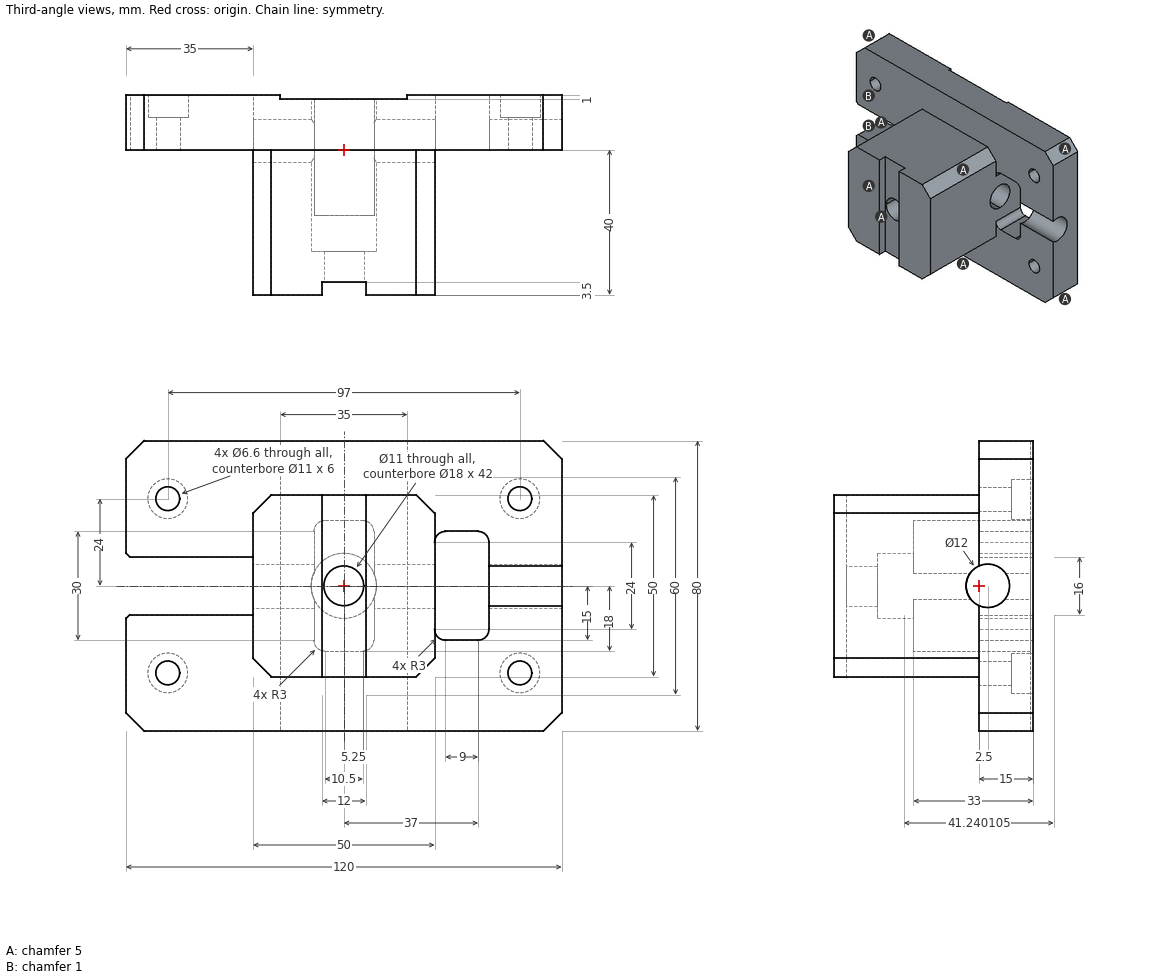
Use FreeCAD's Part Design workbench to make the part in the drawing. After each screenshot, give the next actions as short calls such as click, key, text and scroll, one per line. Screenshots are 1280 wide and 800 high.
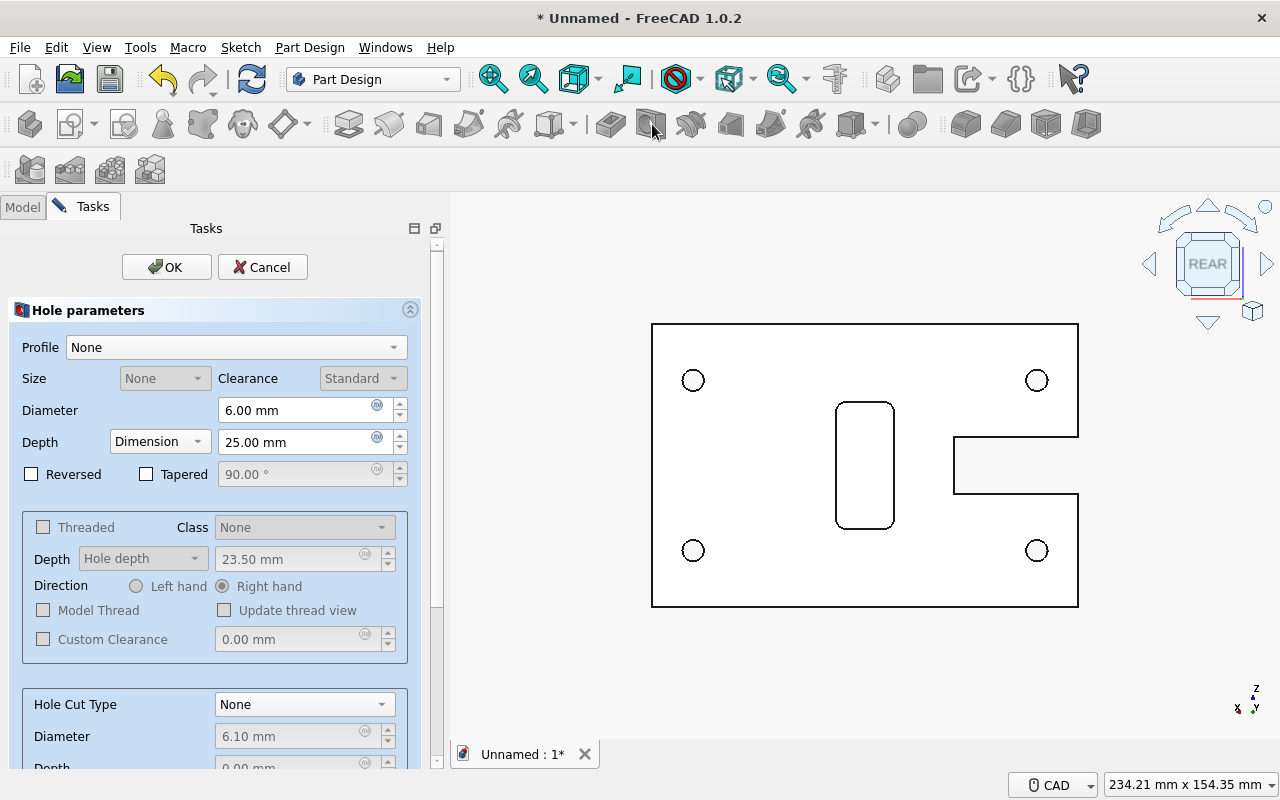
triple_click(305, 410)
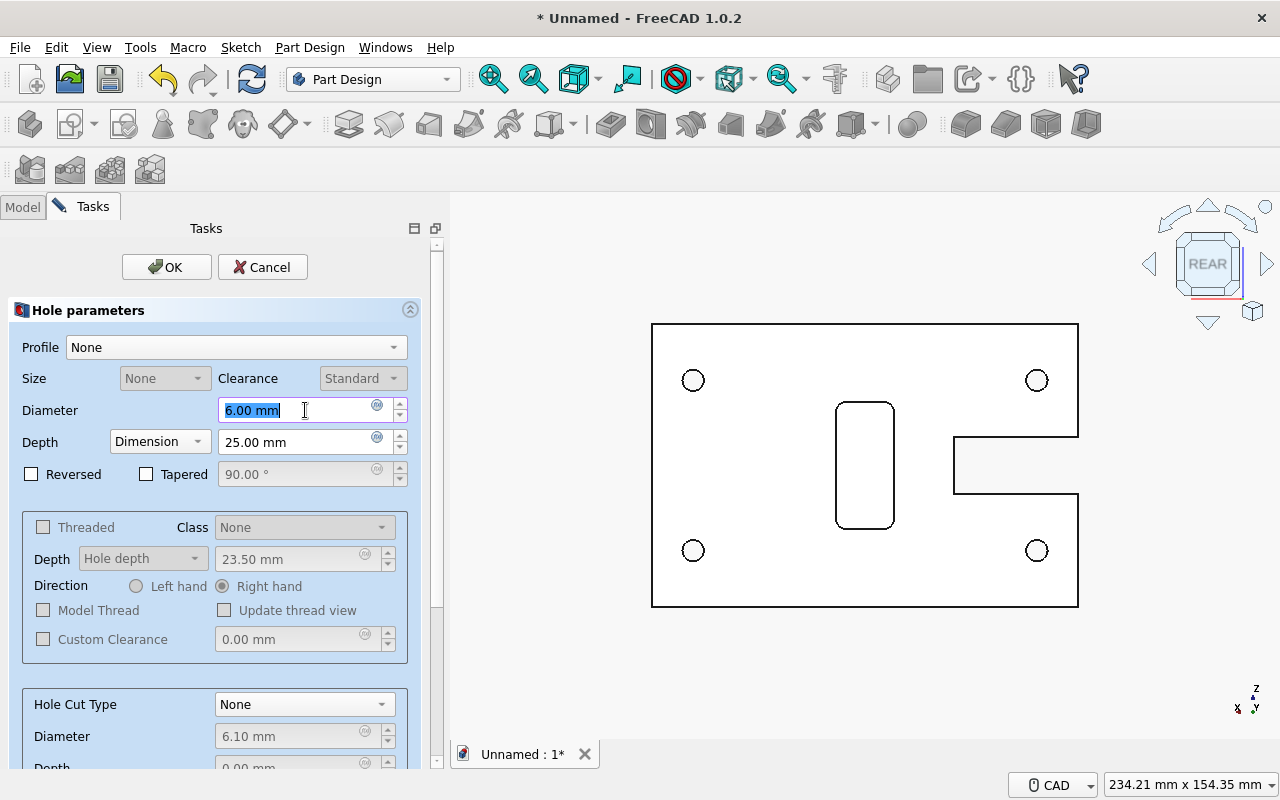
text(6.6)
key(Tab)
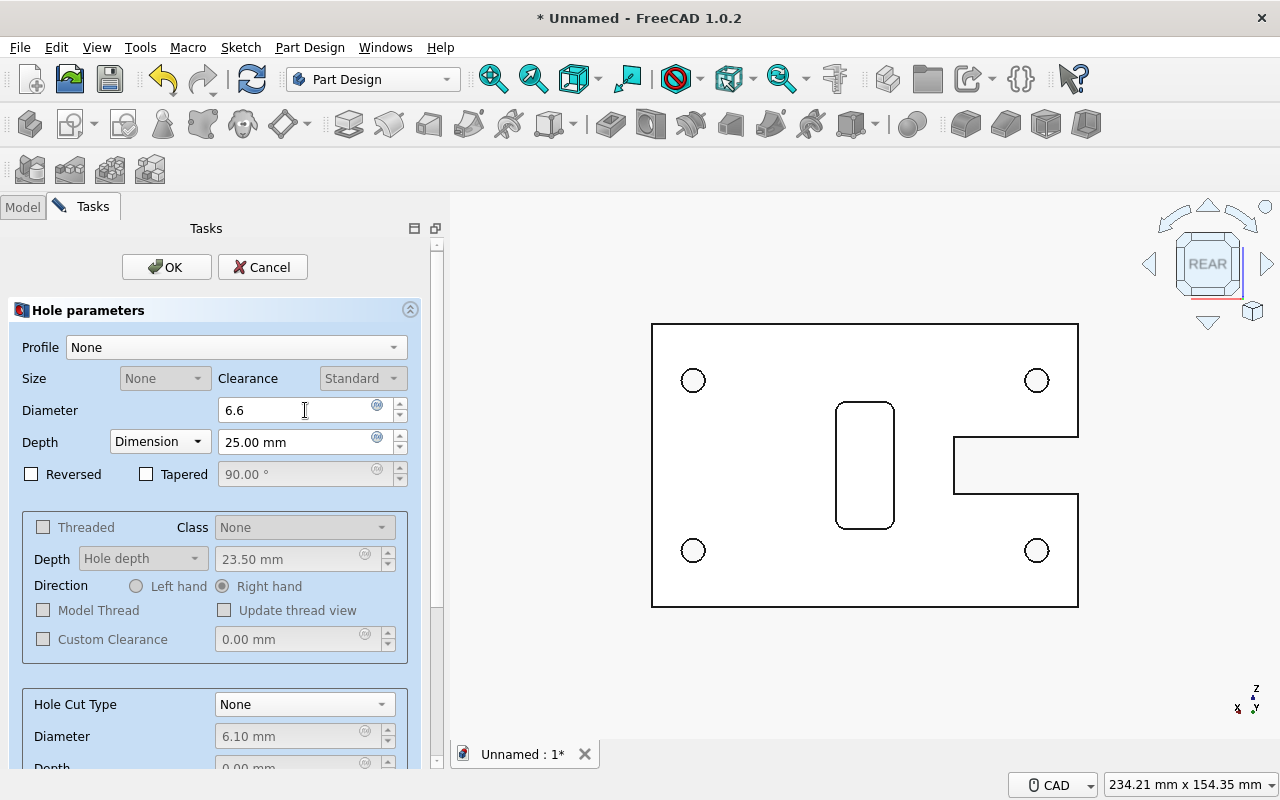
click(161, 442)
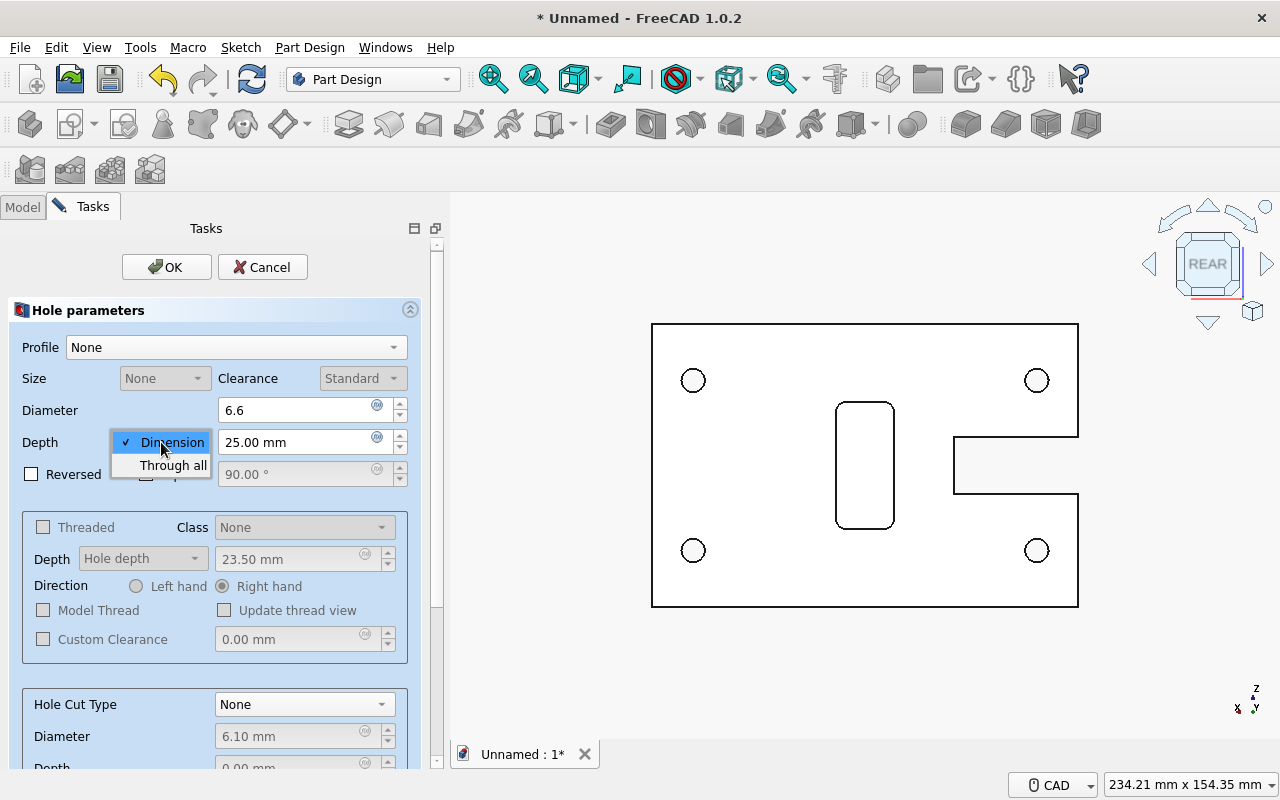
click(160, 466)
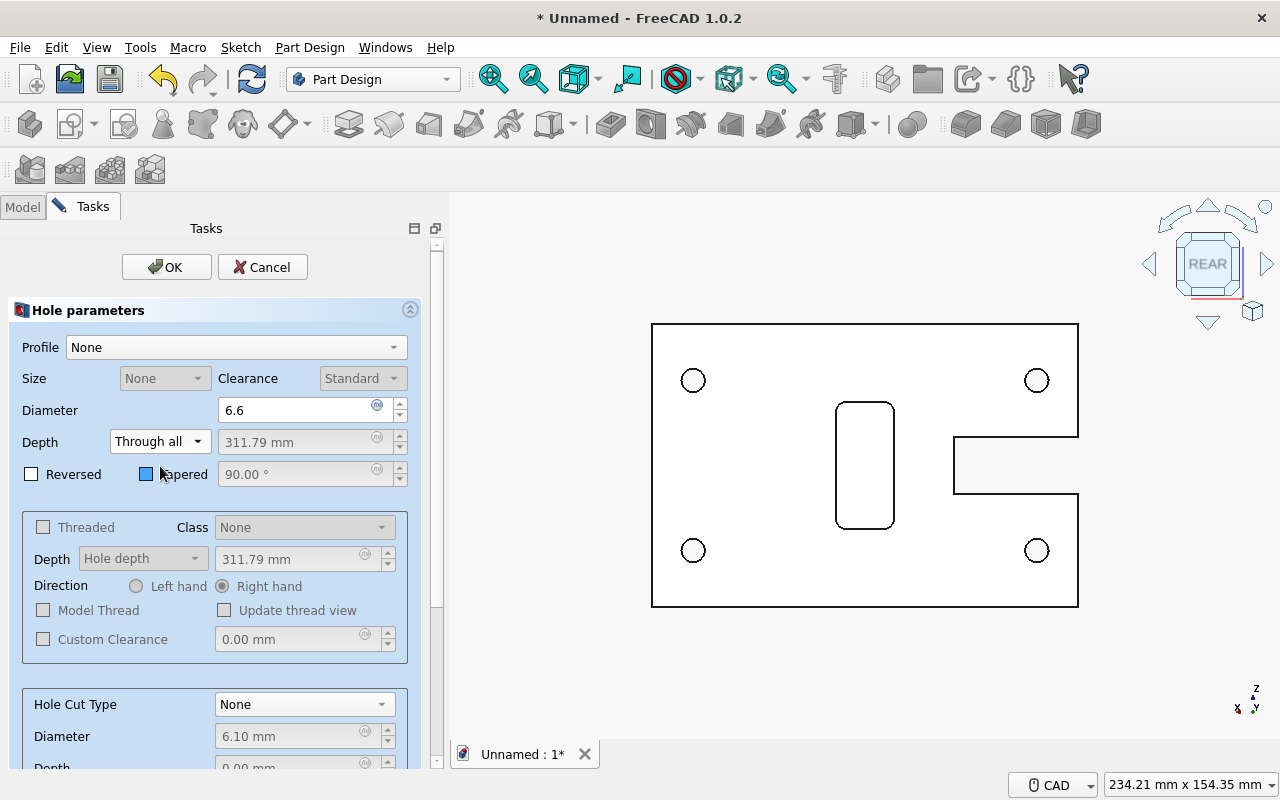
click(306, 704)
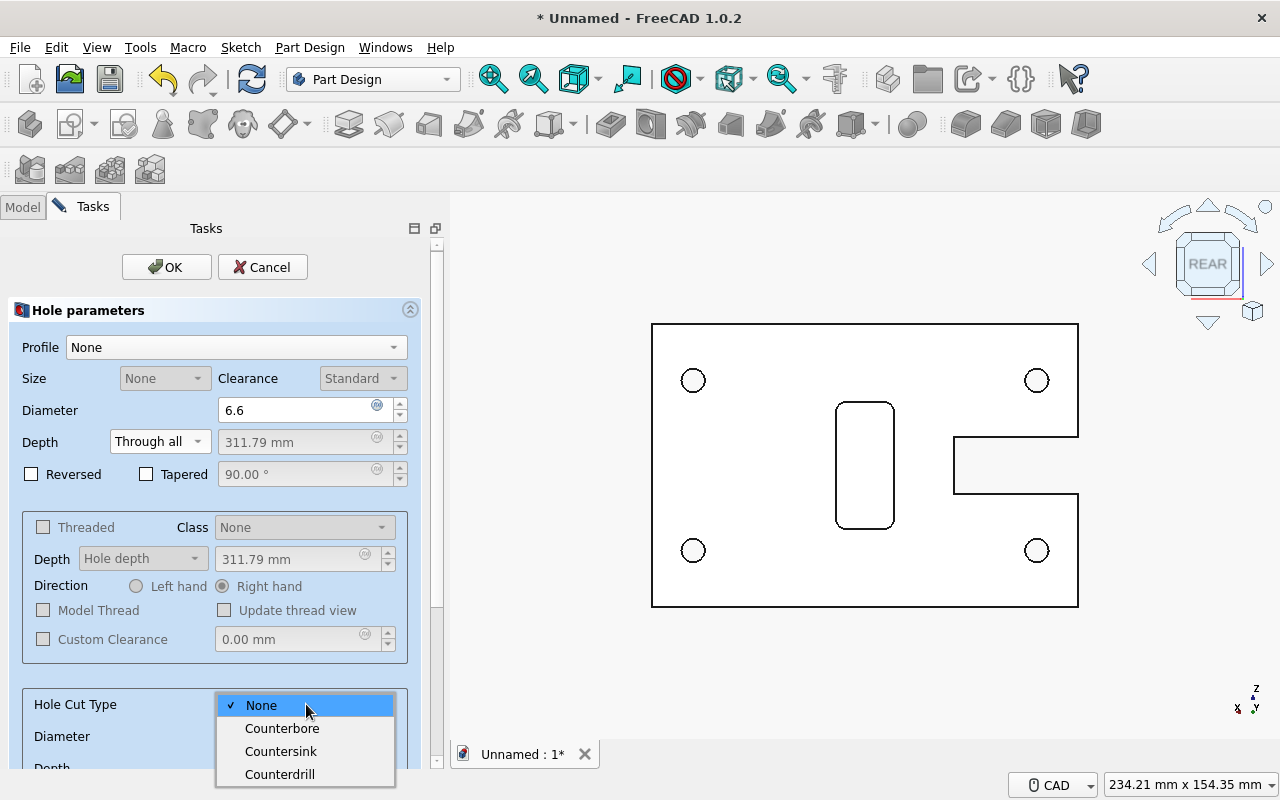
click(304, 728)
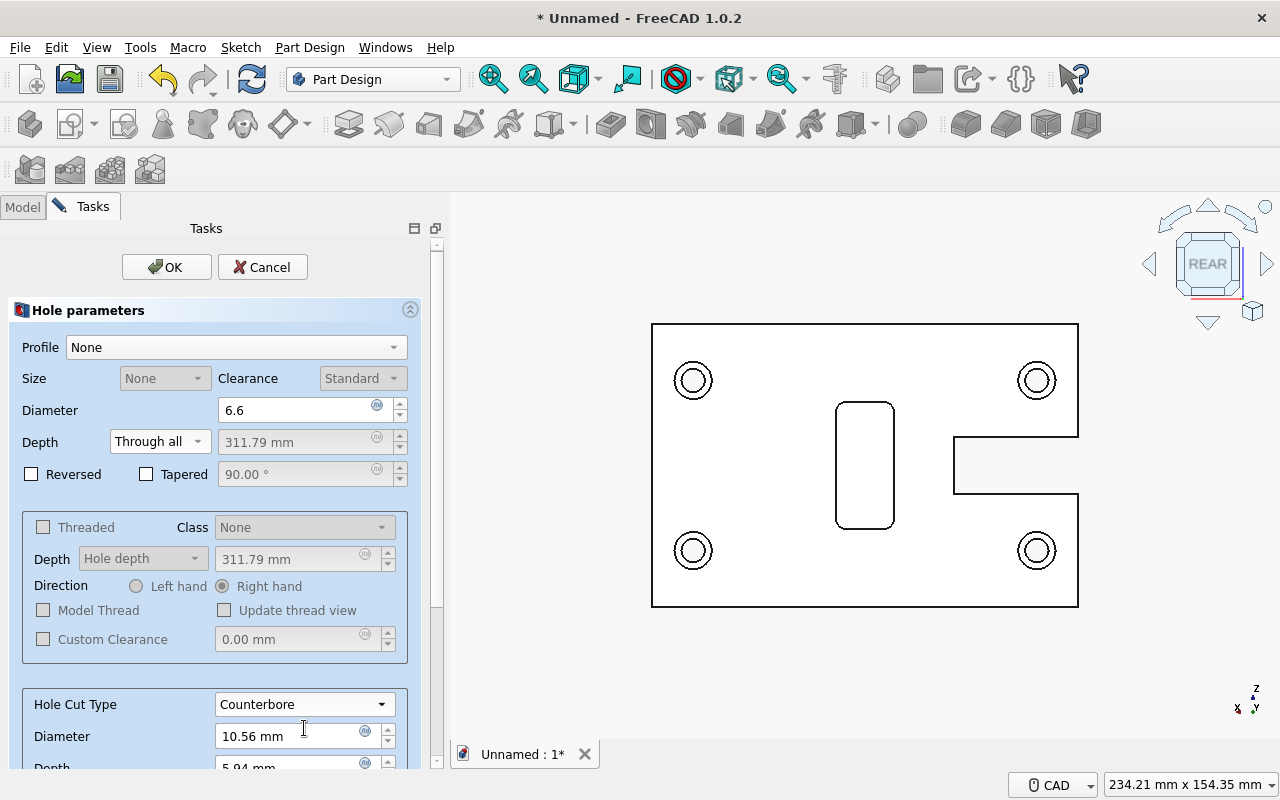
triple_click(298, 736)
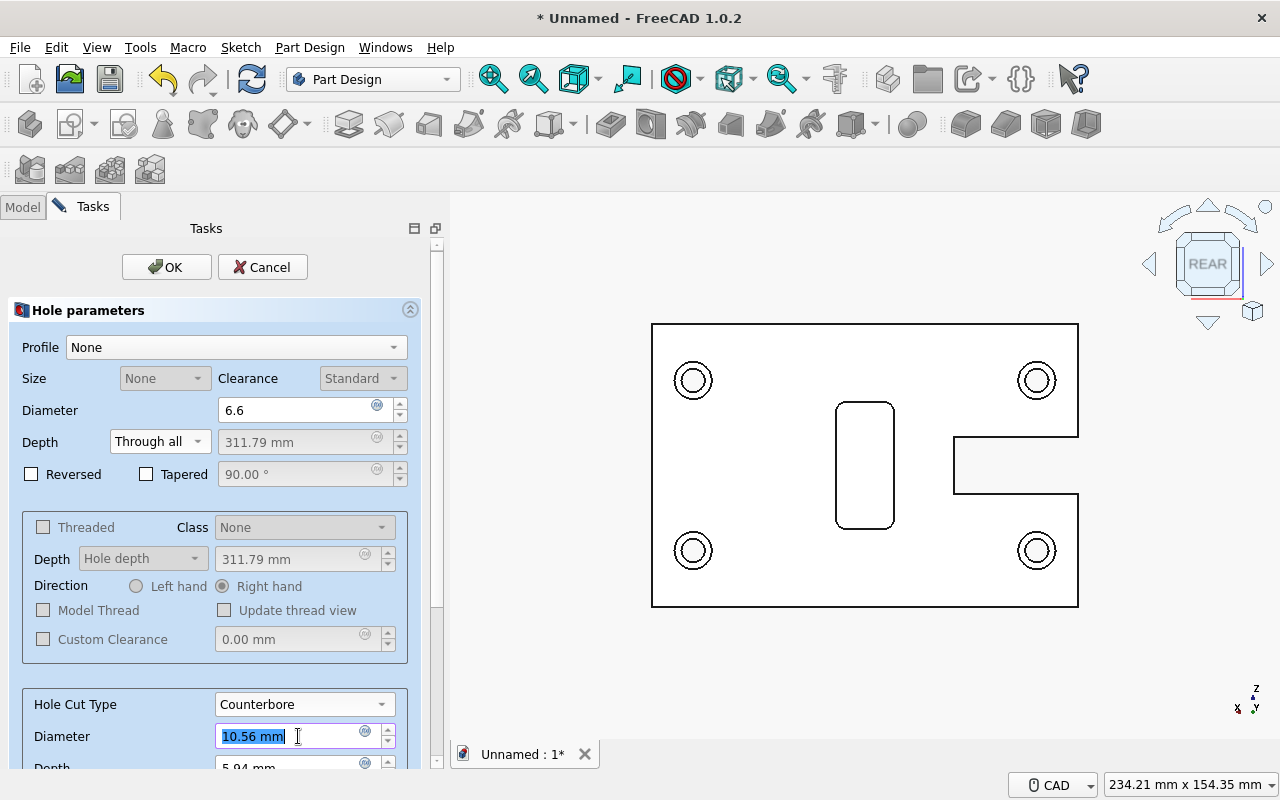
text(11)
key(Tab)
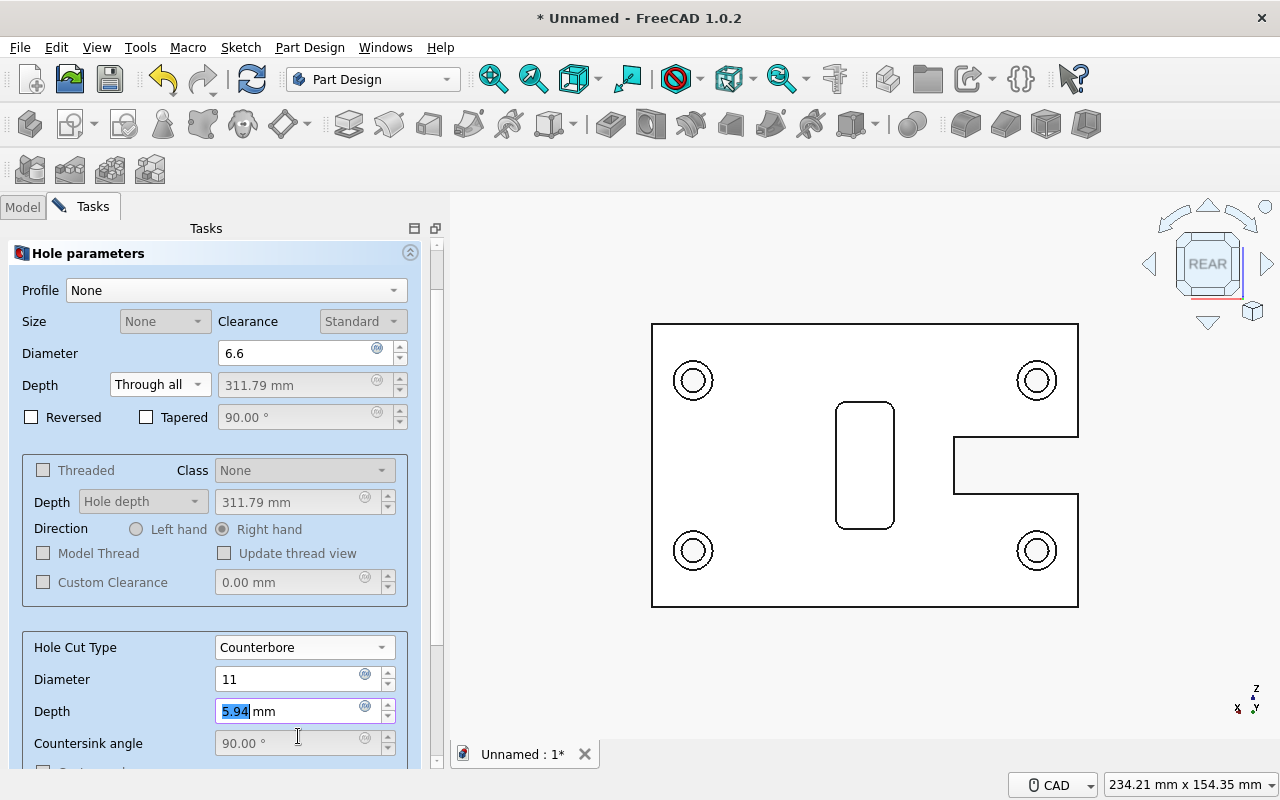
text(6)
key(Tab)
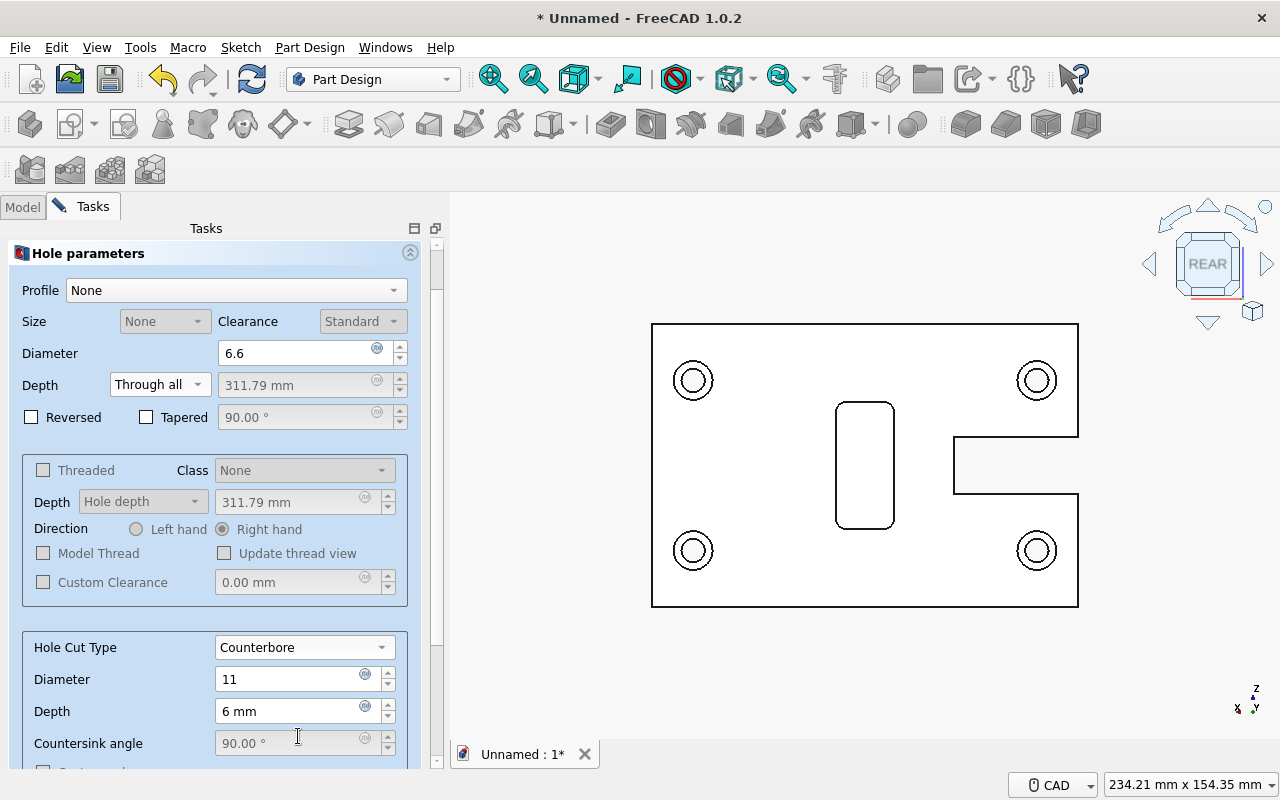
scroll(437, 503, up, 2)